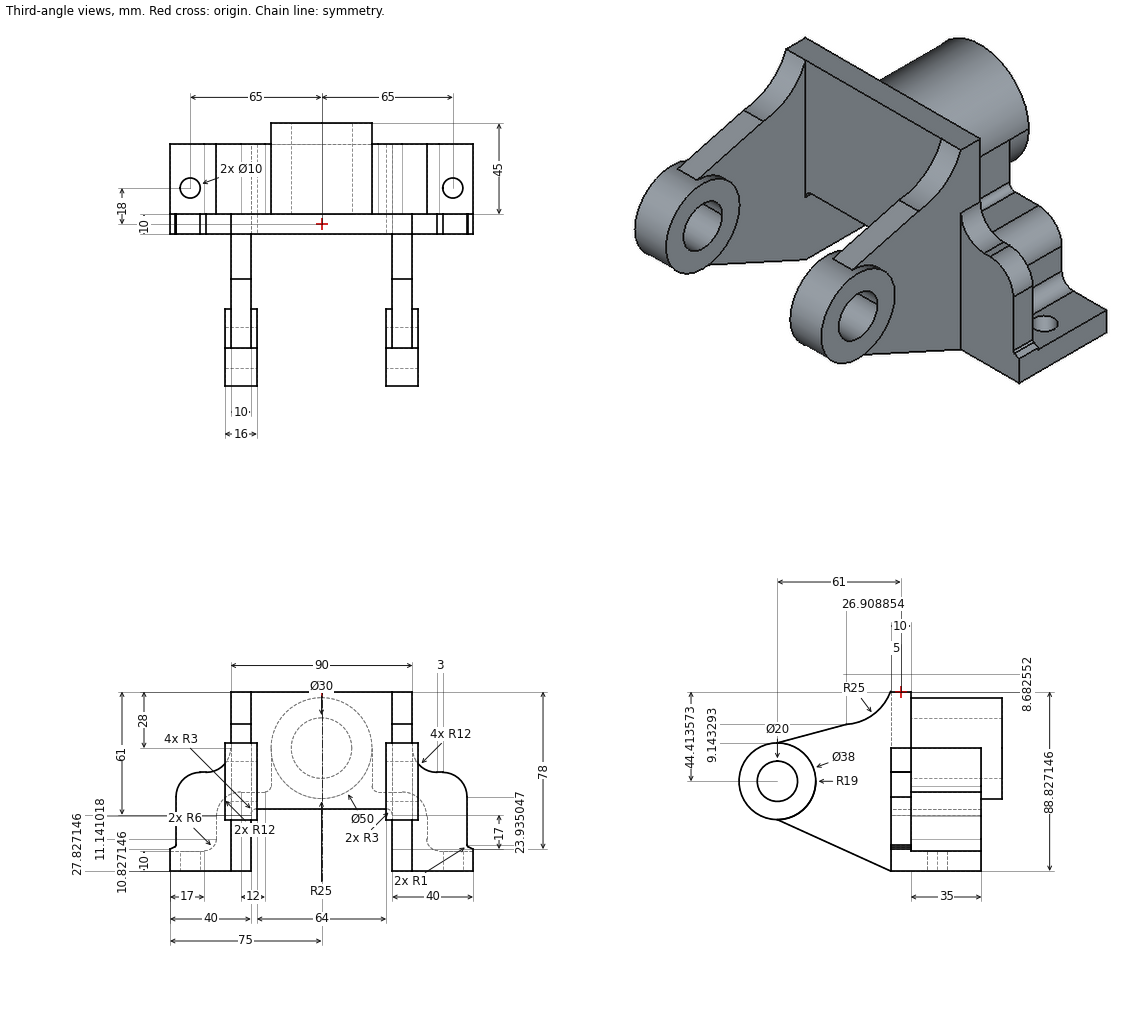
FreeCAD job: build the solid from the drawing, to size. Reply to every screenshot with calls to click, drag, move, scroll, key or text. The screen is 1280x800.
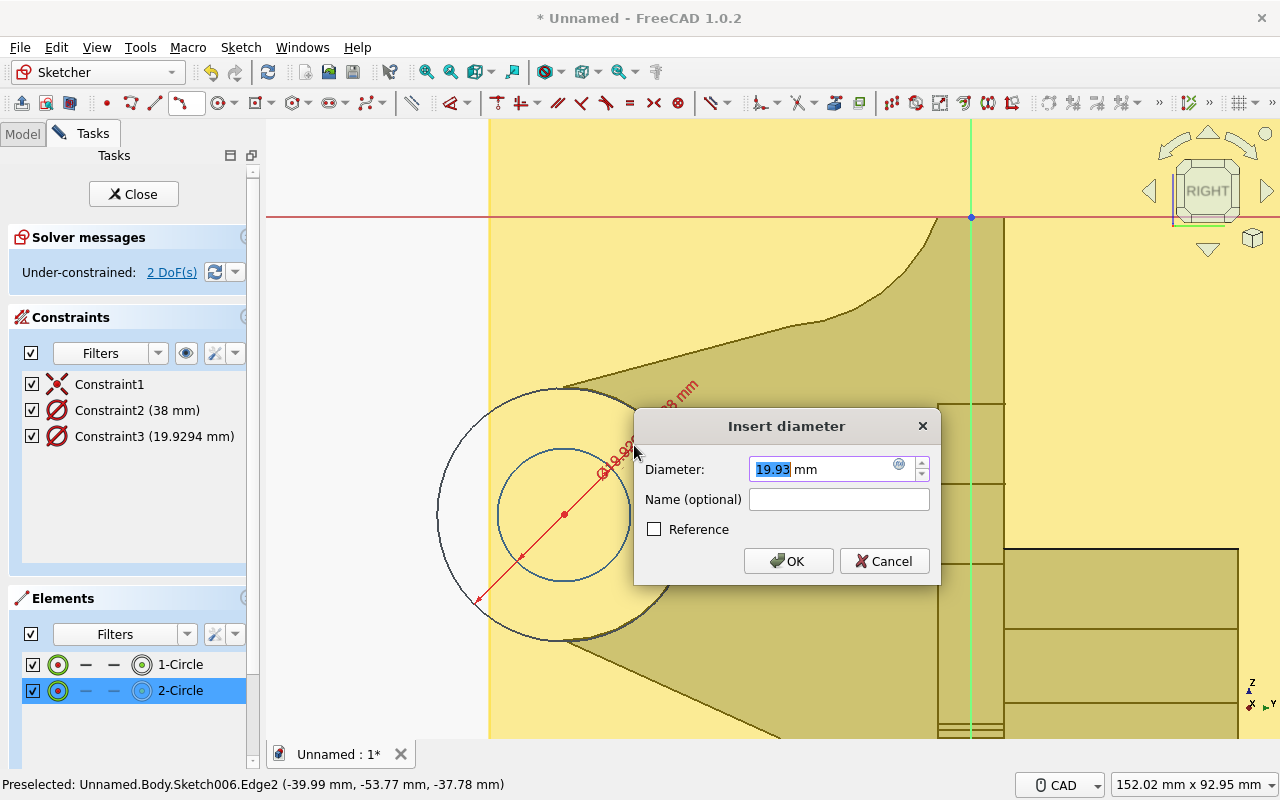
text(20)
key(Return)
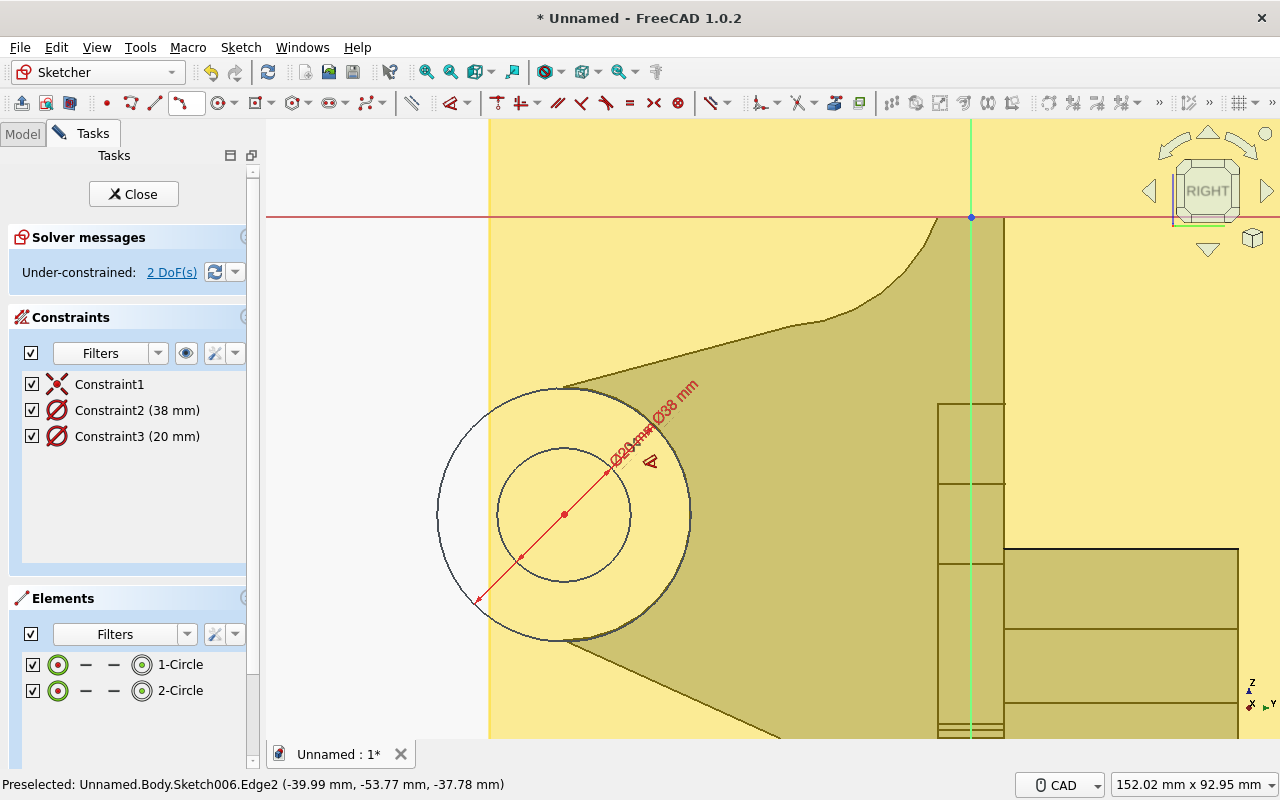
click(564, 515)
click(768, 183)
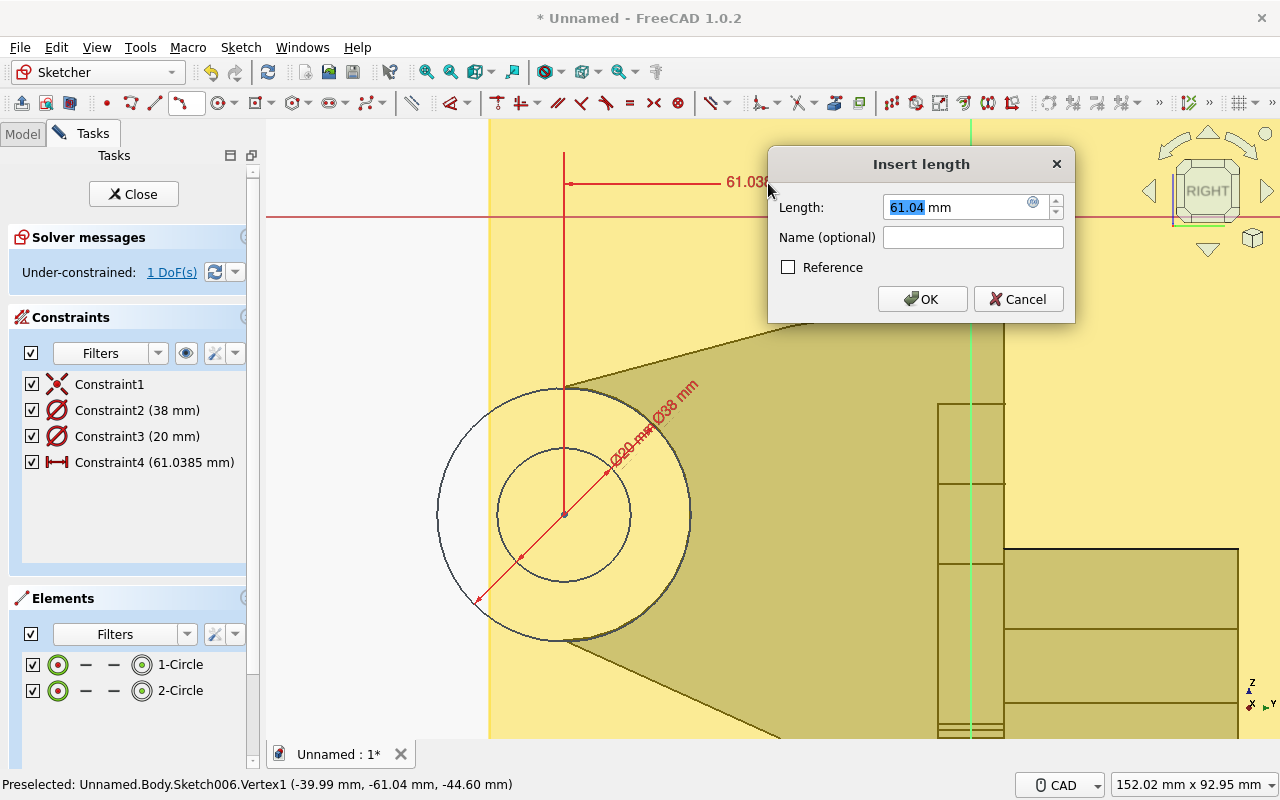
text(61)
key(Return)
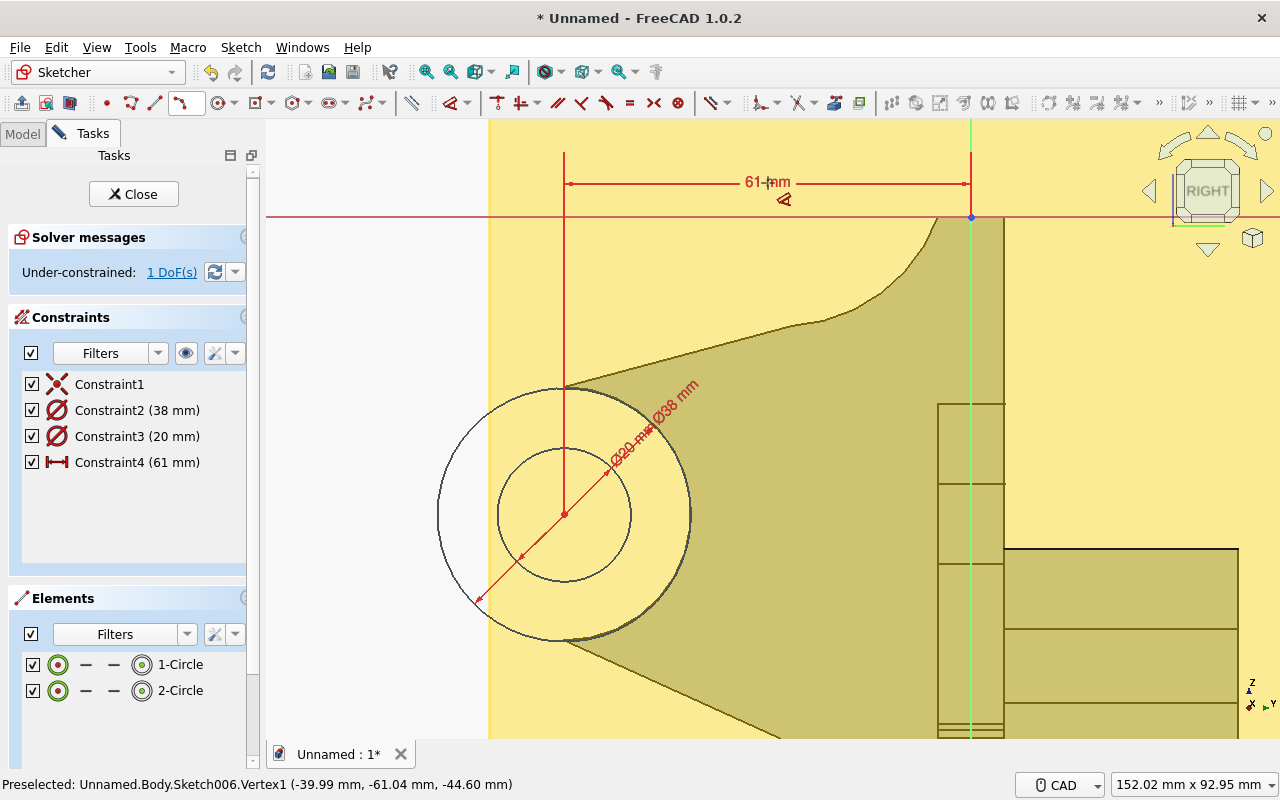
click(564, 515)
click(1005, 366)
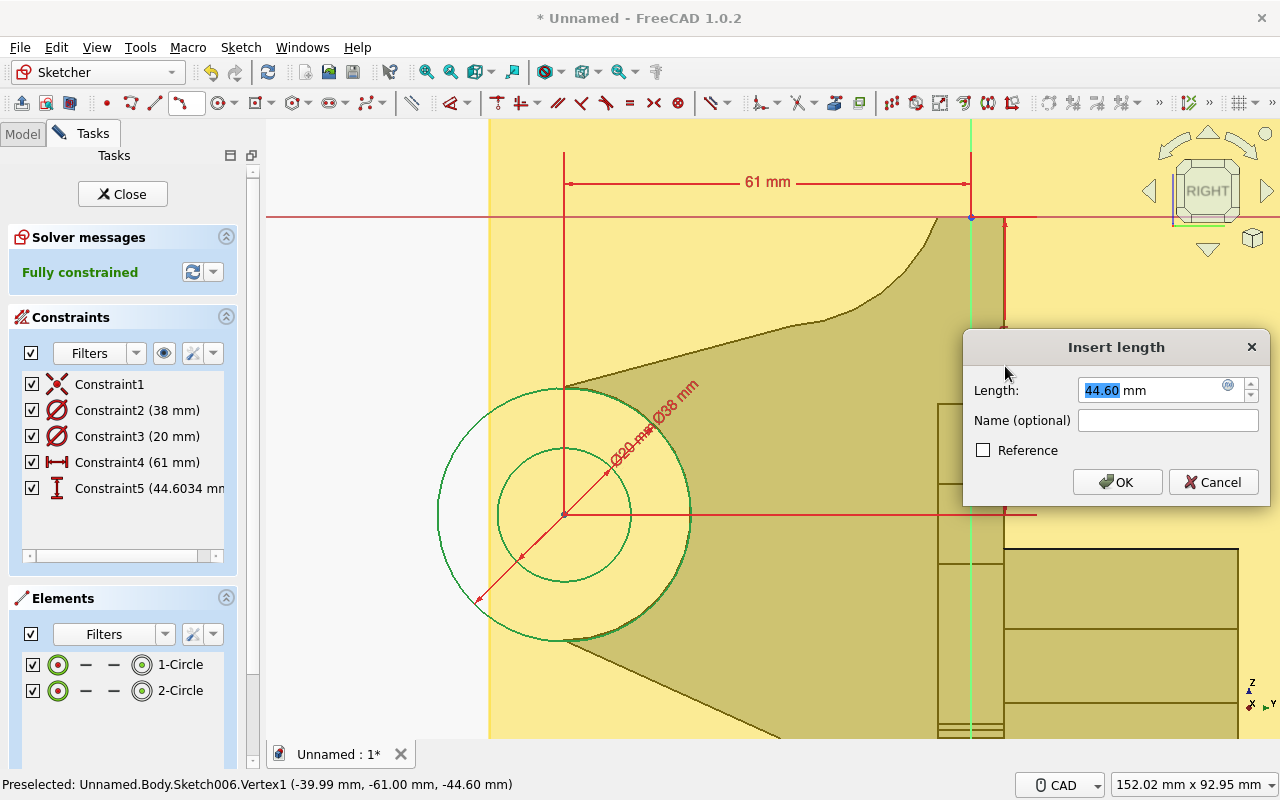
text(44.413573)
key(Return)
key(Escape)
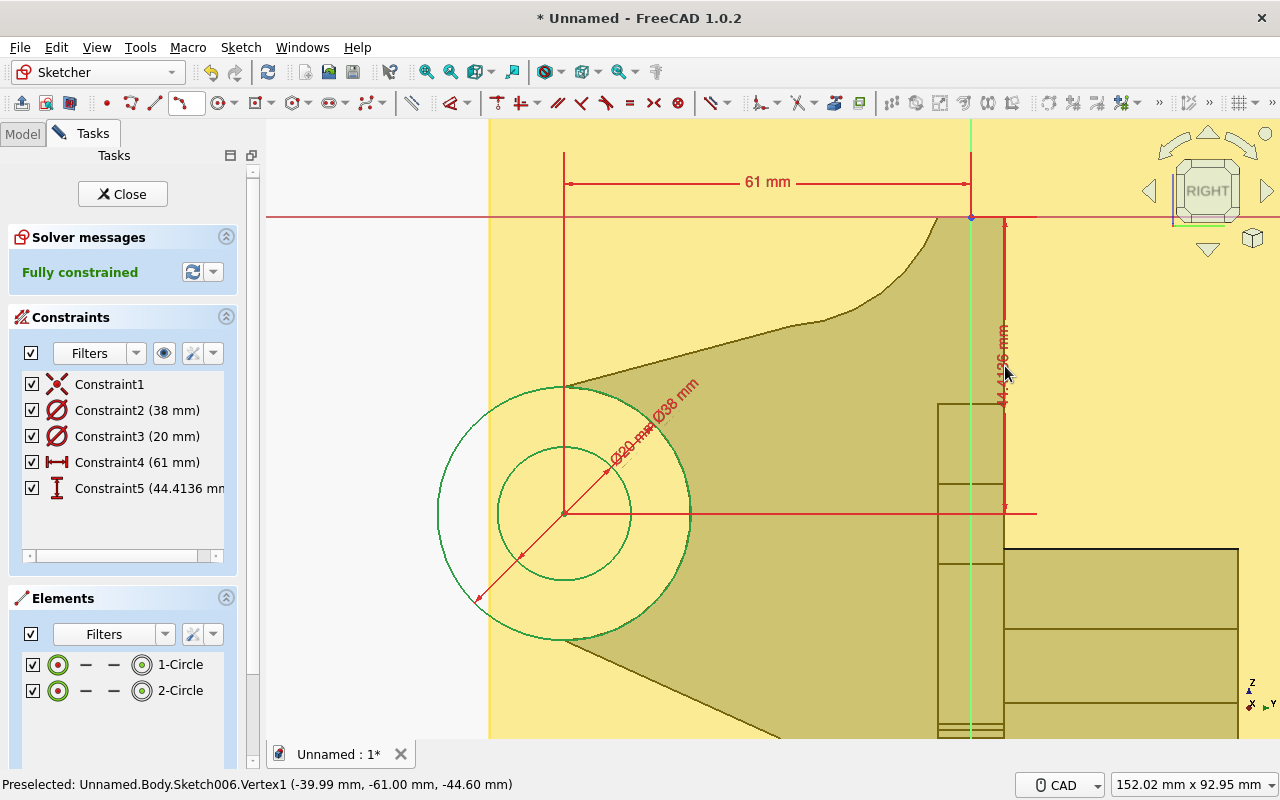
click(123, 194)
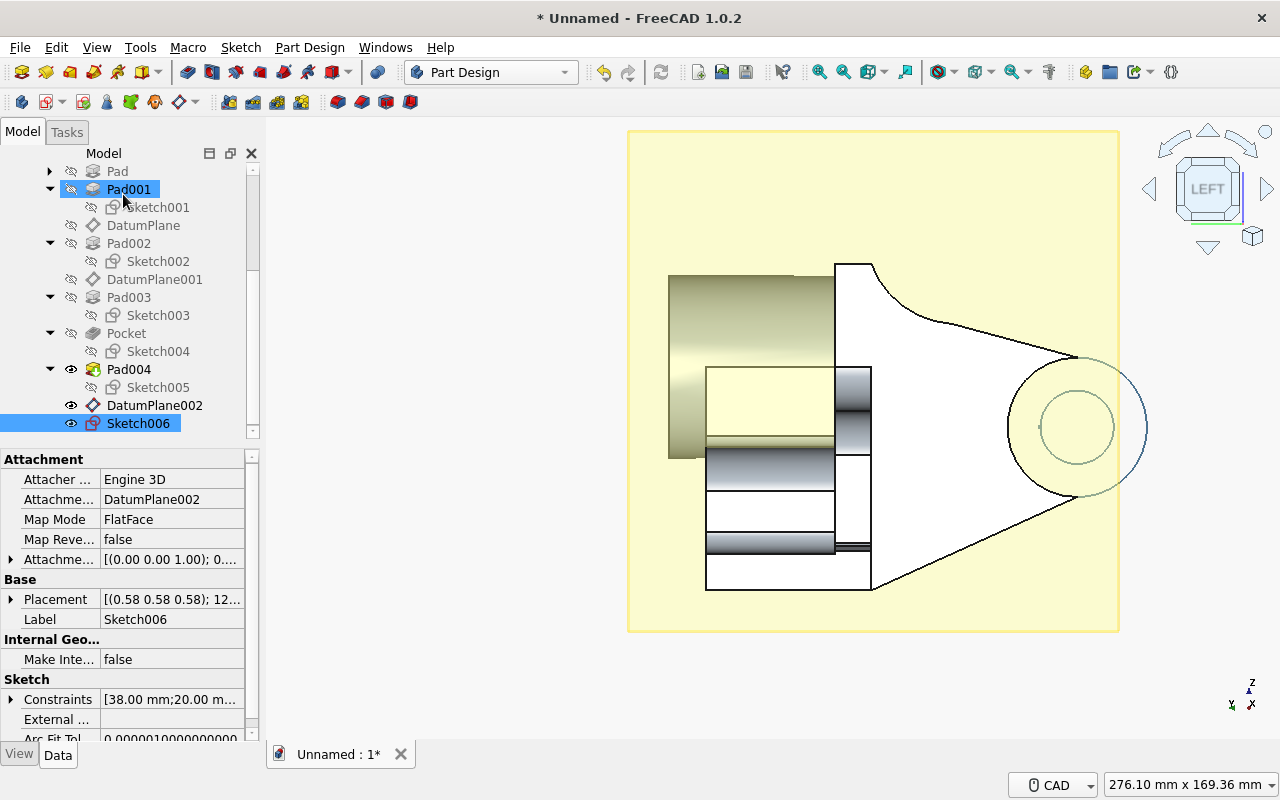
click(22, 72)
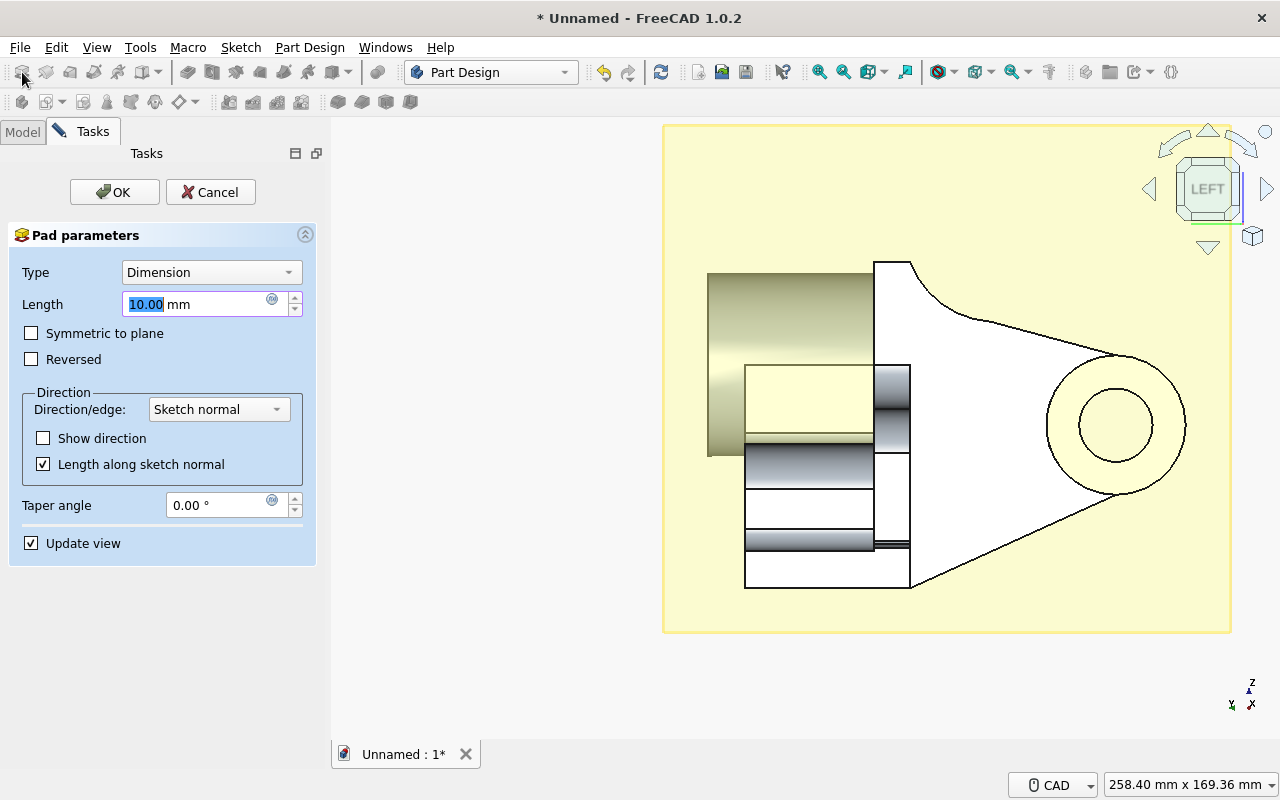
text(16)
key(Tab)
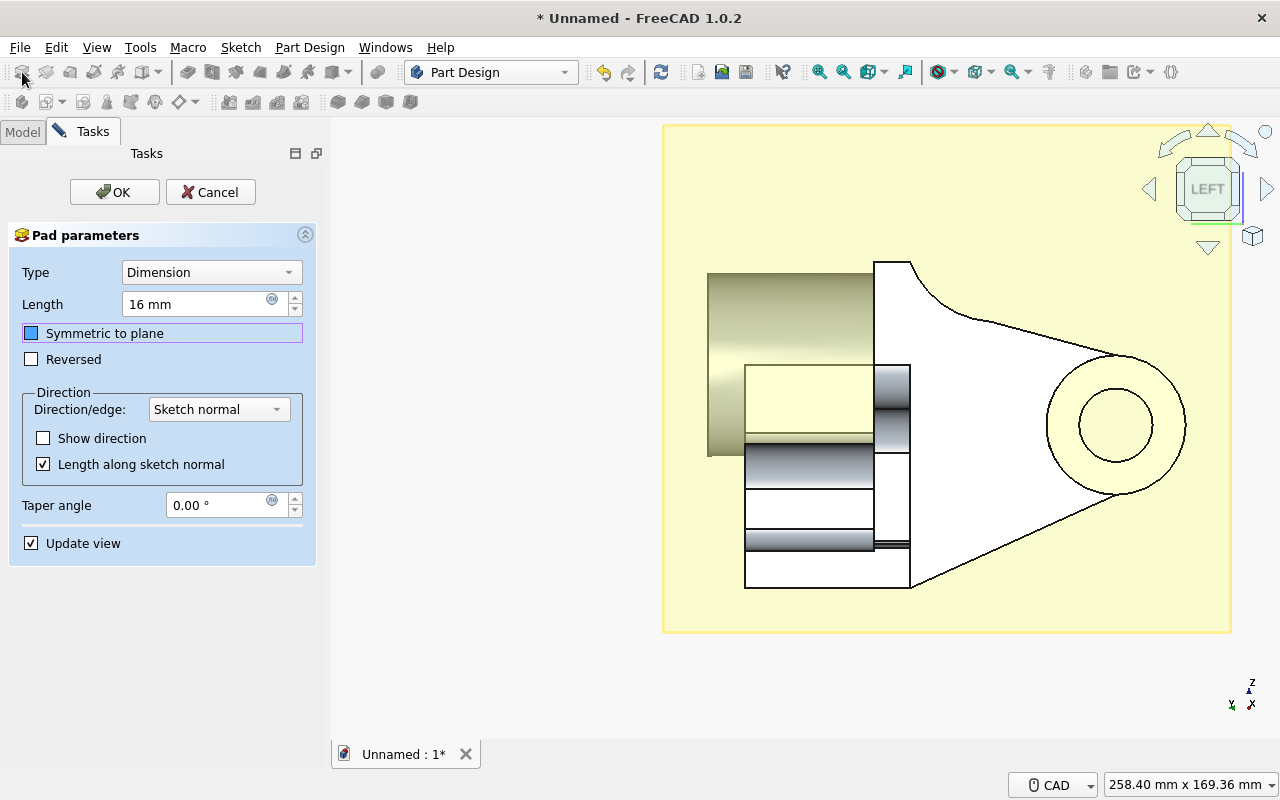
click(30, 333)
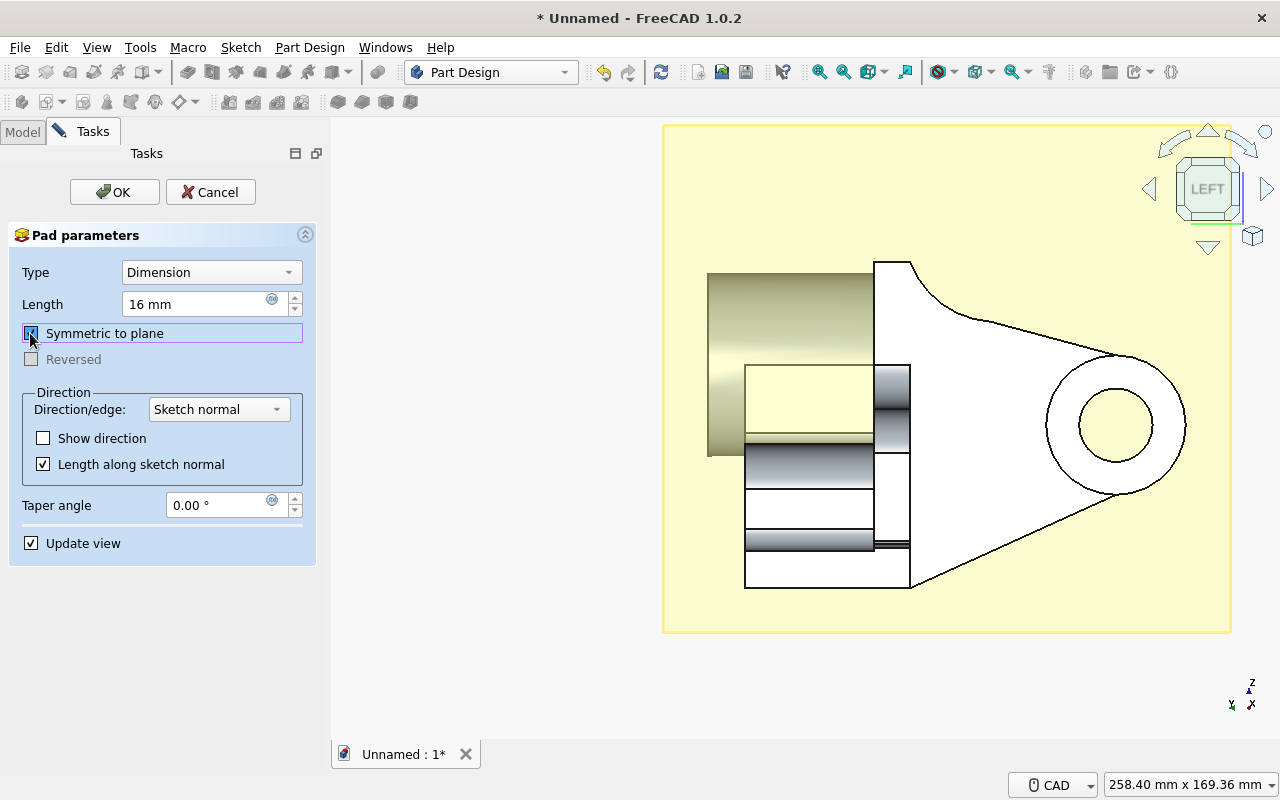
click(115, 192)